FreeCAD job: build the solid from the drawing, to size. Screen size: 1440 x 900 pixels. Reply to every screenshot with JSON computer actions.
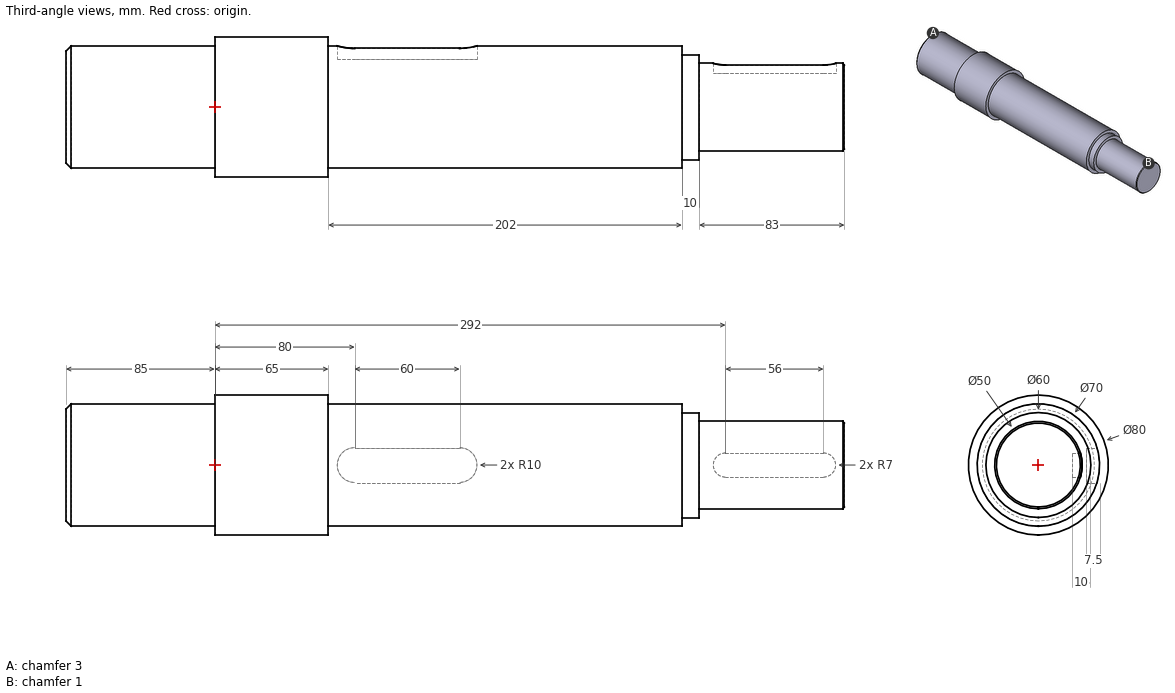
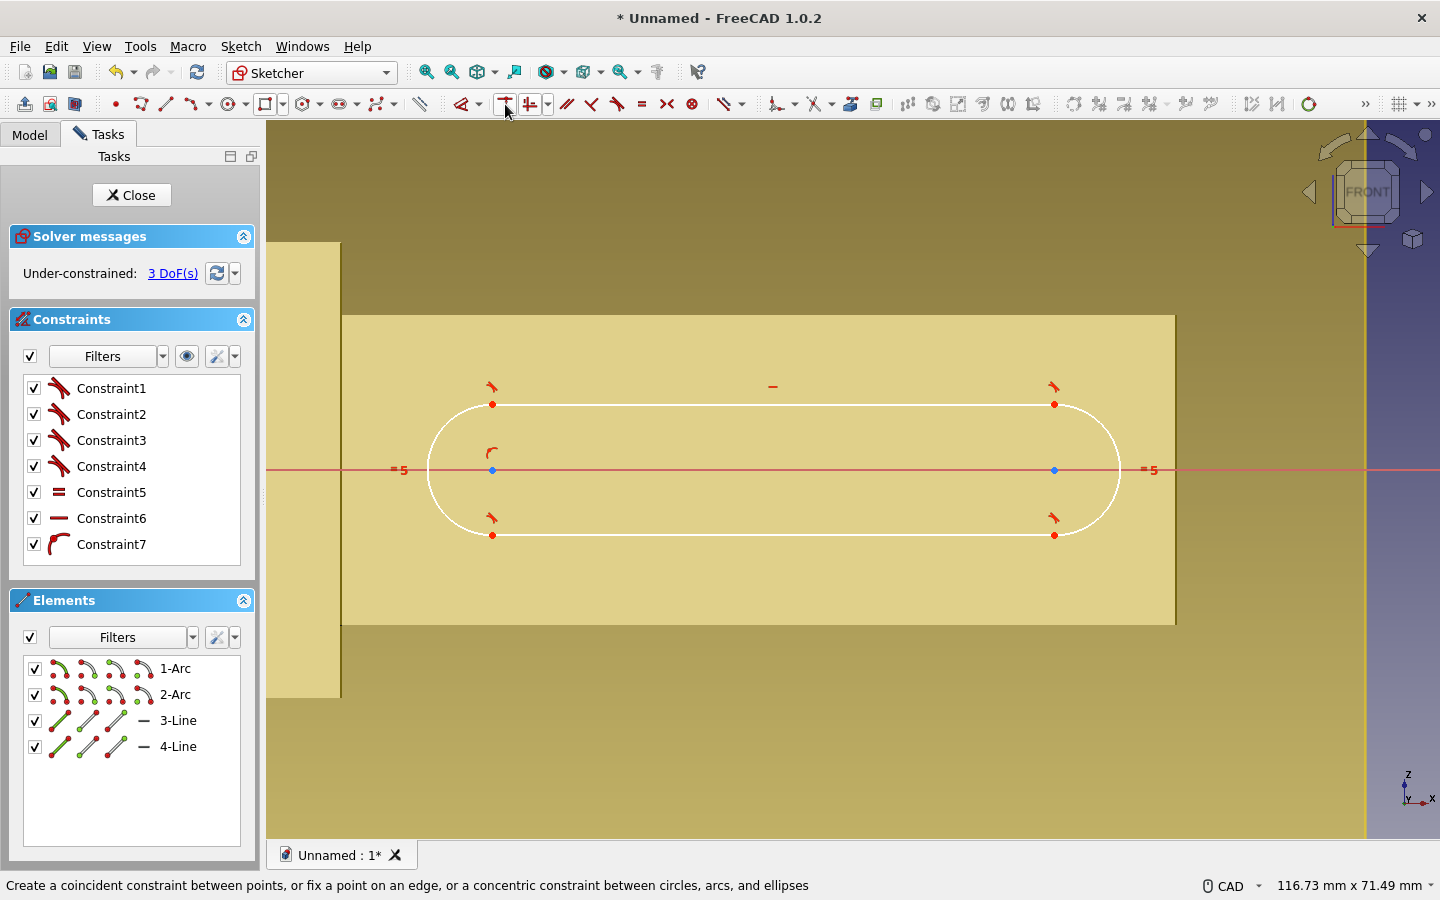
{"action": "left_click", "coordinate": [440, 432]}
{"action": "left_click", "coordinate": [414, 413]}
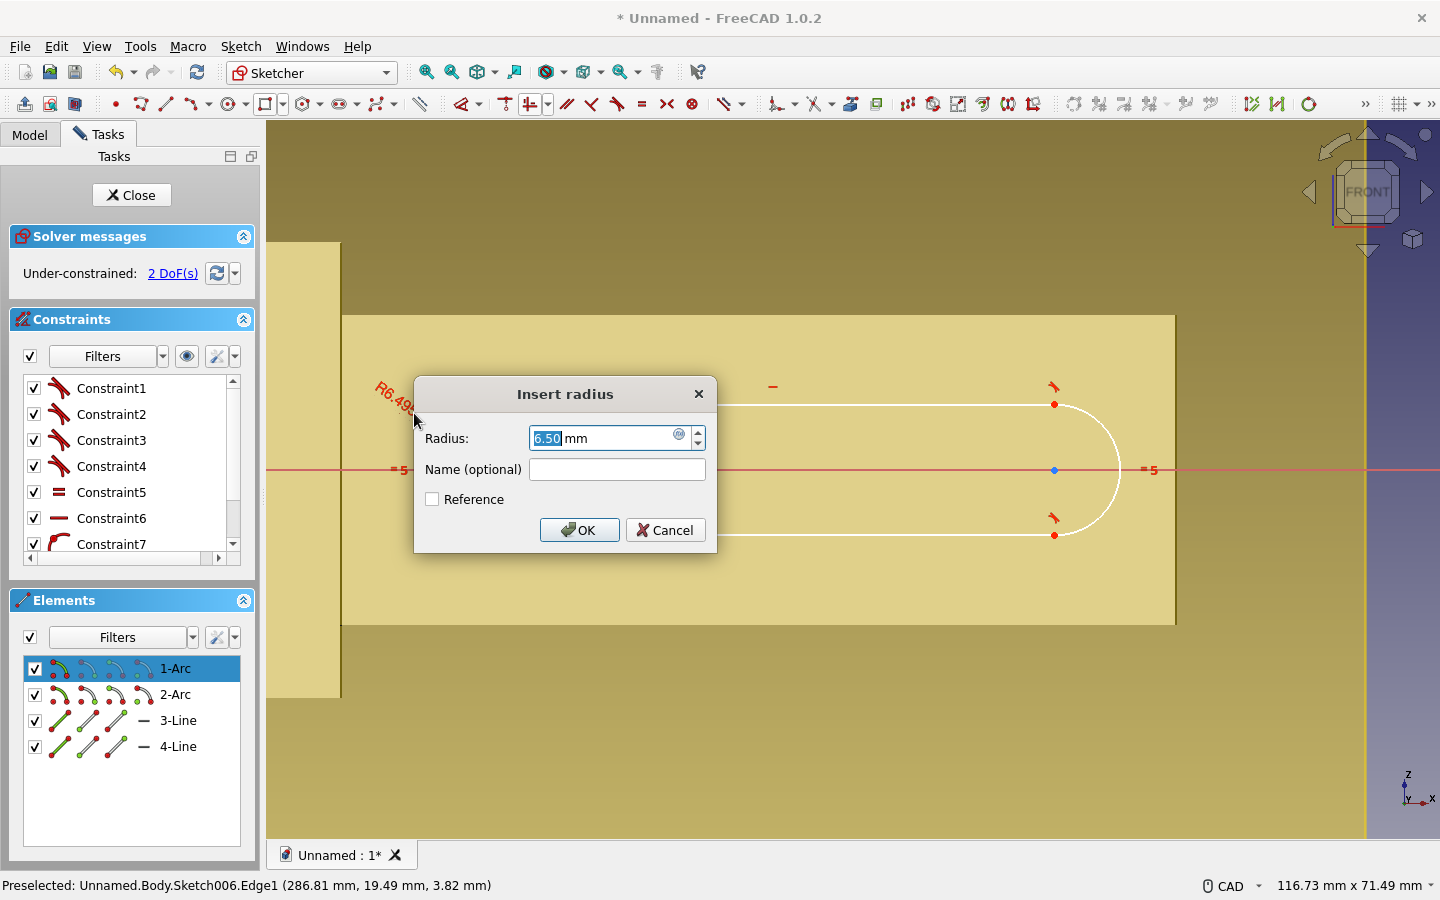
{"action": "type", "text": "7"}
{"action": "key", "text": "Return"}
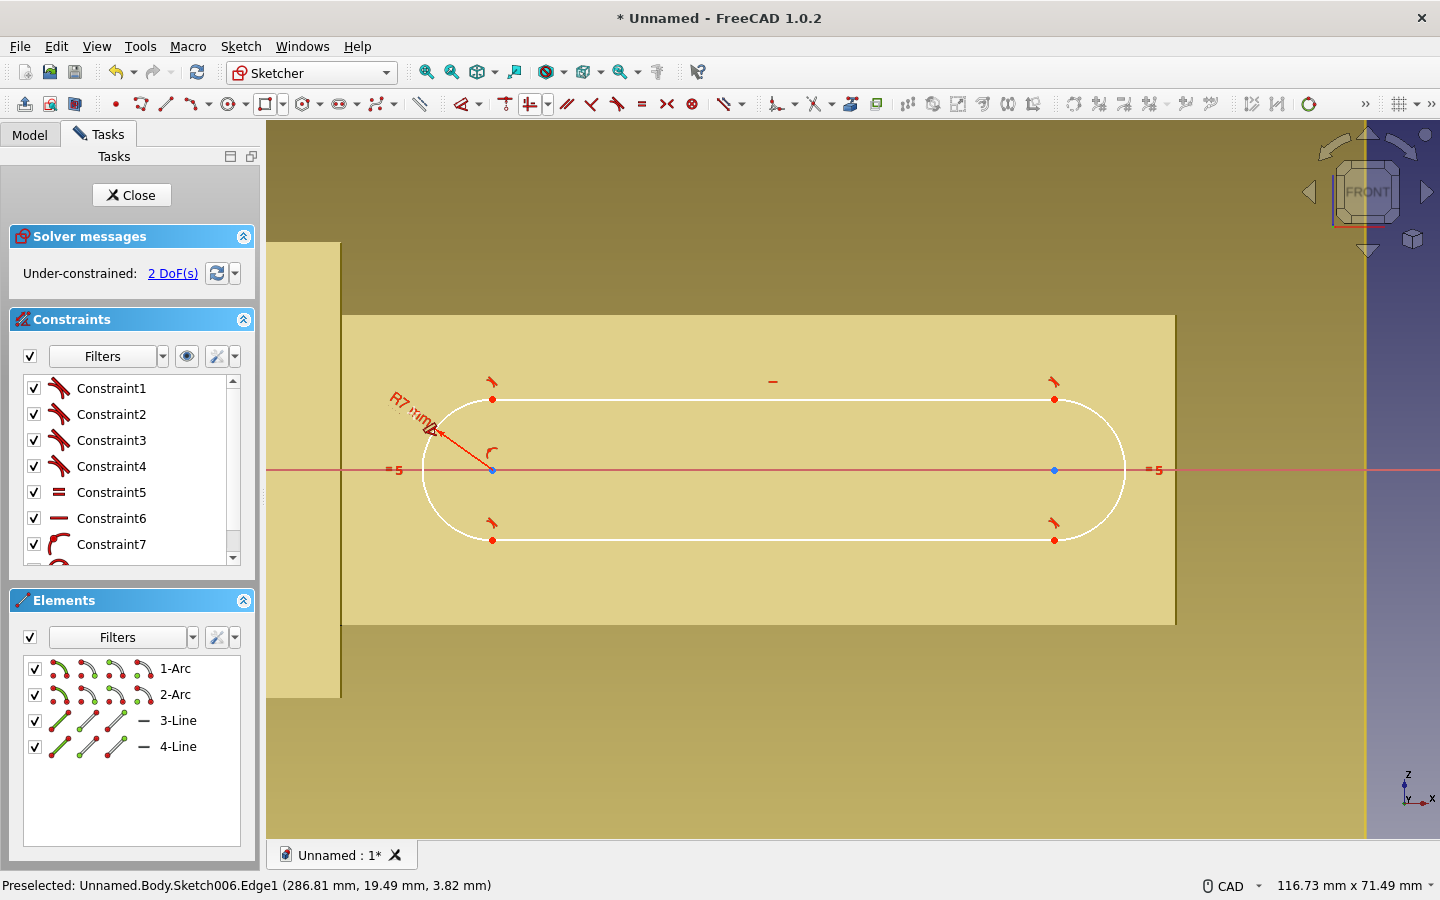
{"action": "left_click", "coordinate": [661, 400]}
{"action": "left_click", "coordinate": [774, 366]}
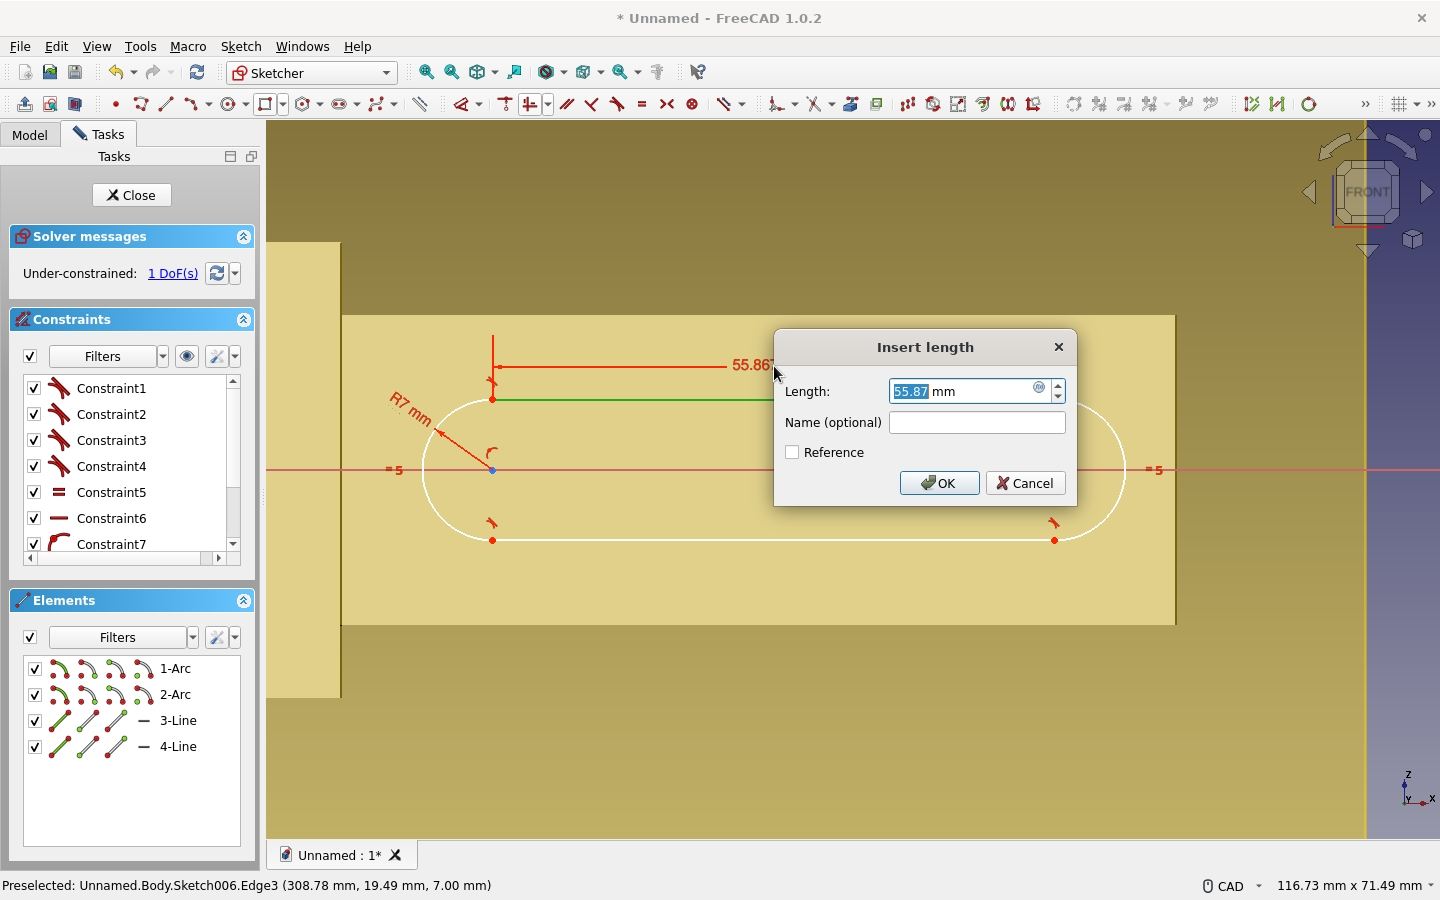
{"action": "type", "text": "56"}
{"action": "key", "text": "Return"}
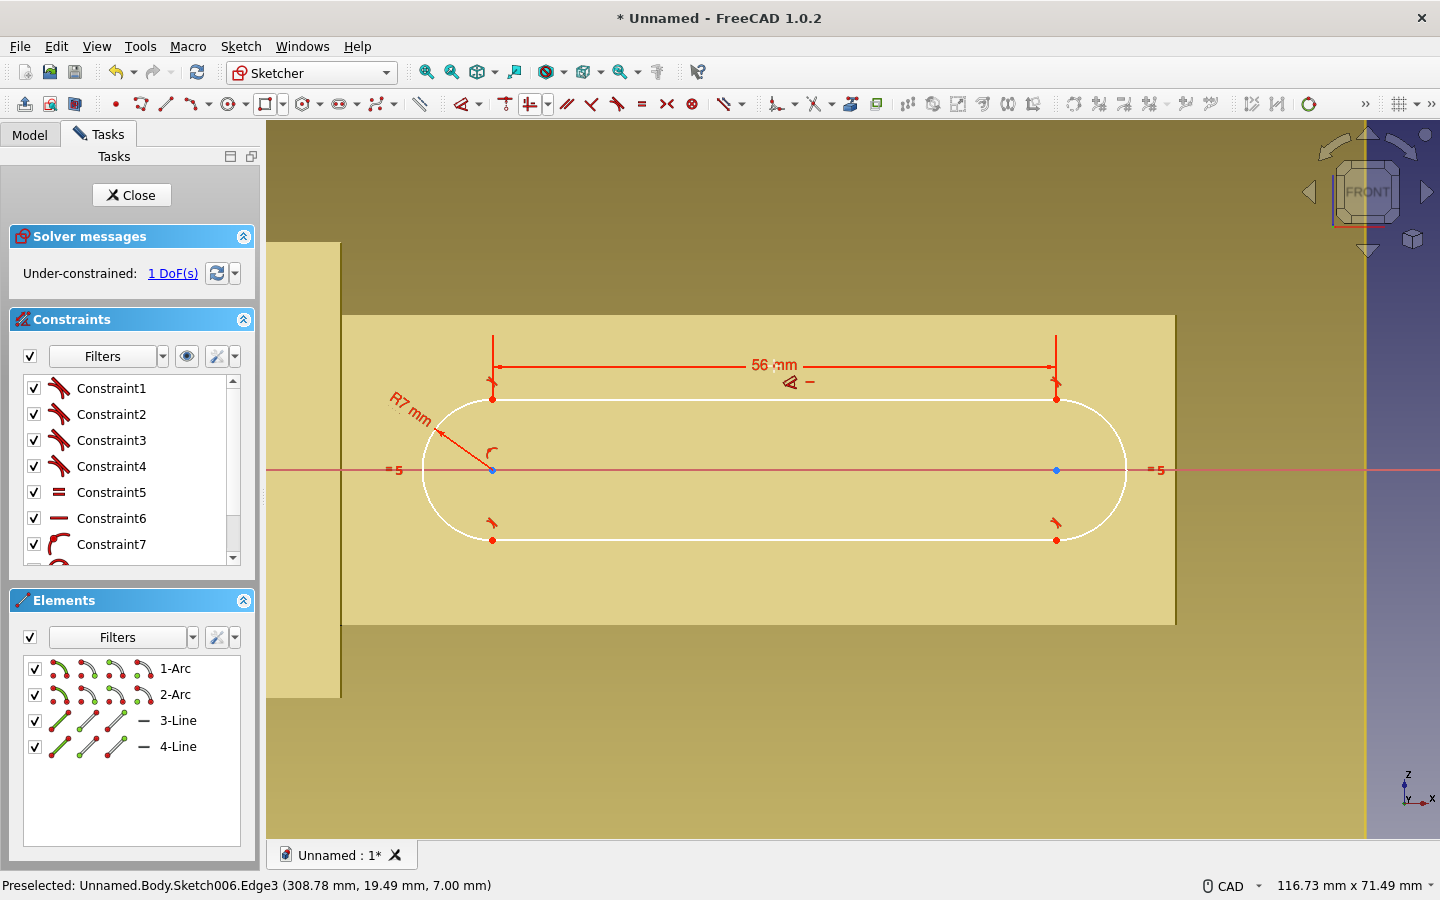
{"action": "left_click", "coordinate": [493, 400]}
{"action": "left_click", "coordinate": [393, 366]}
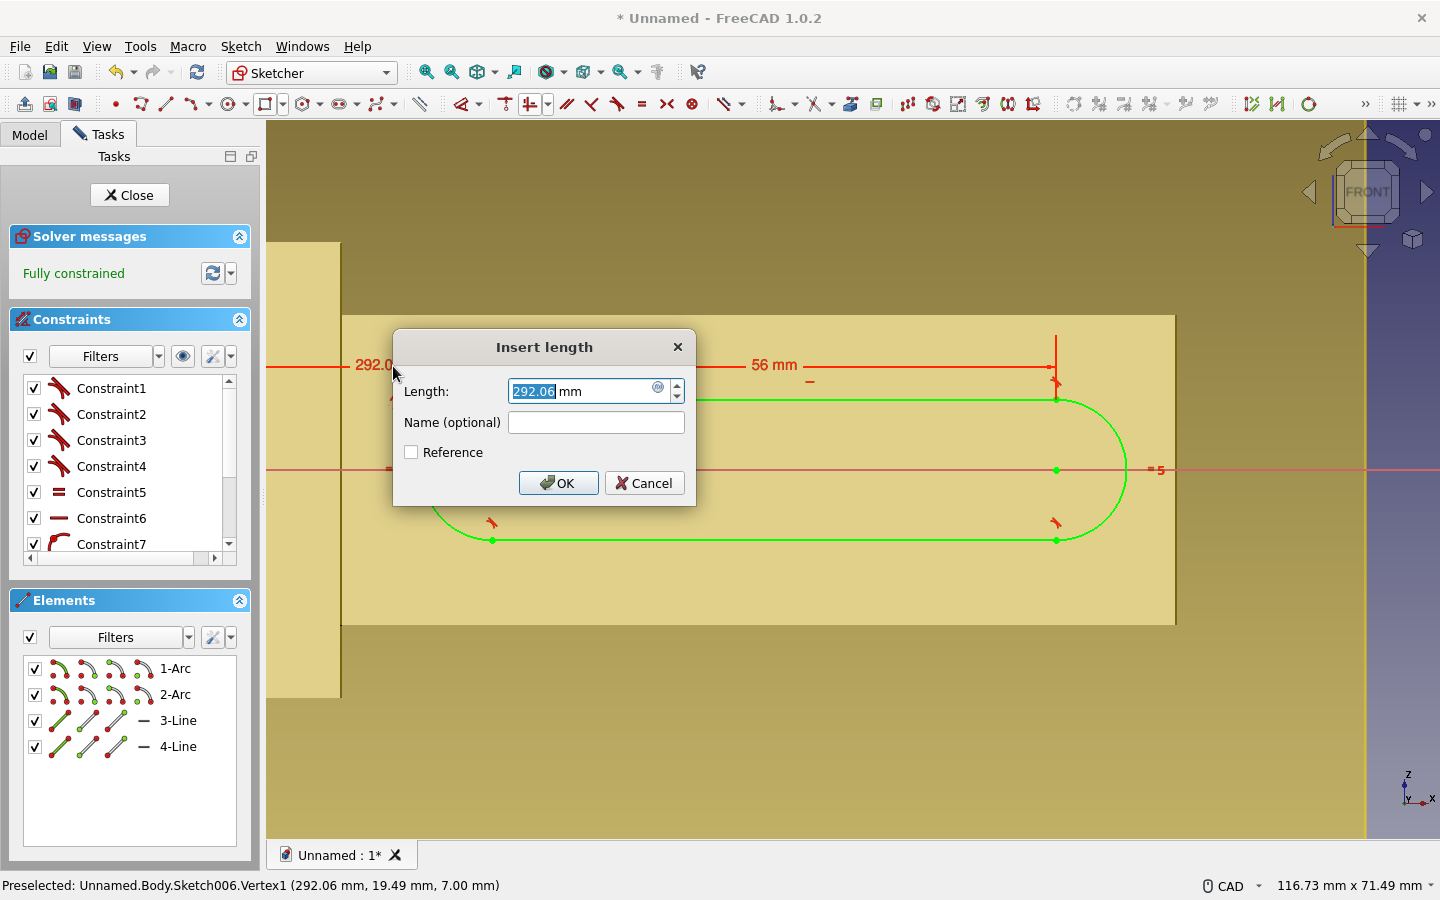
{"action": "type", "text": "292"}
{"action": "key", "text": "Return"}
{"action": "key", "text": "Escape"}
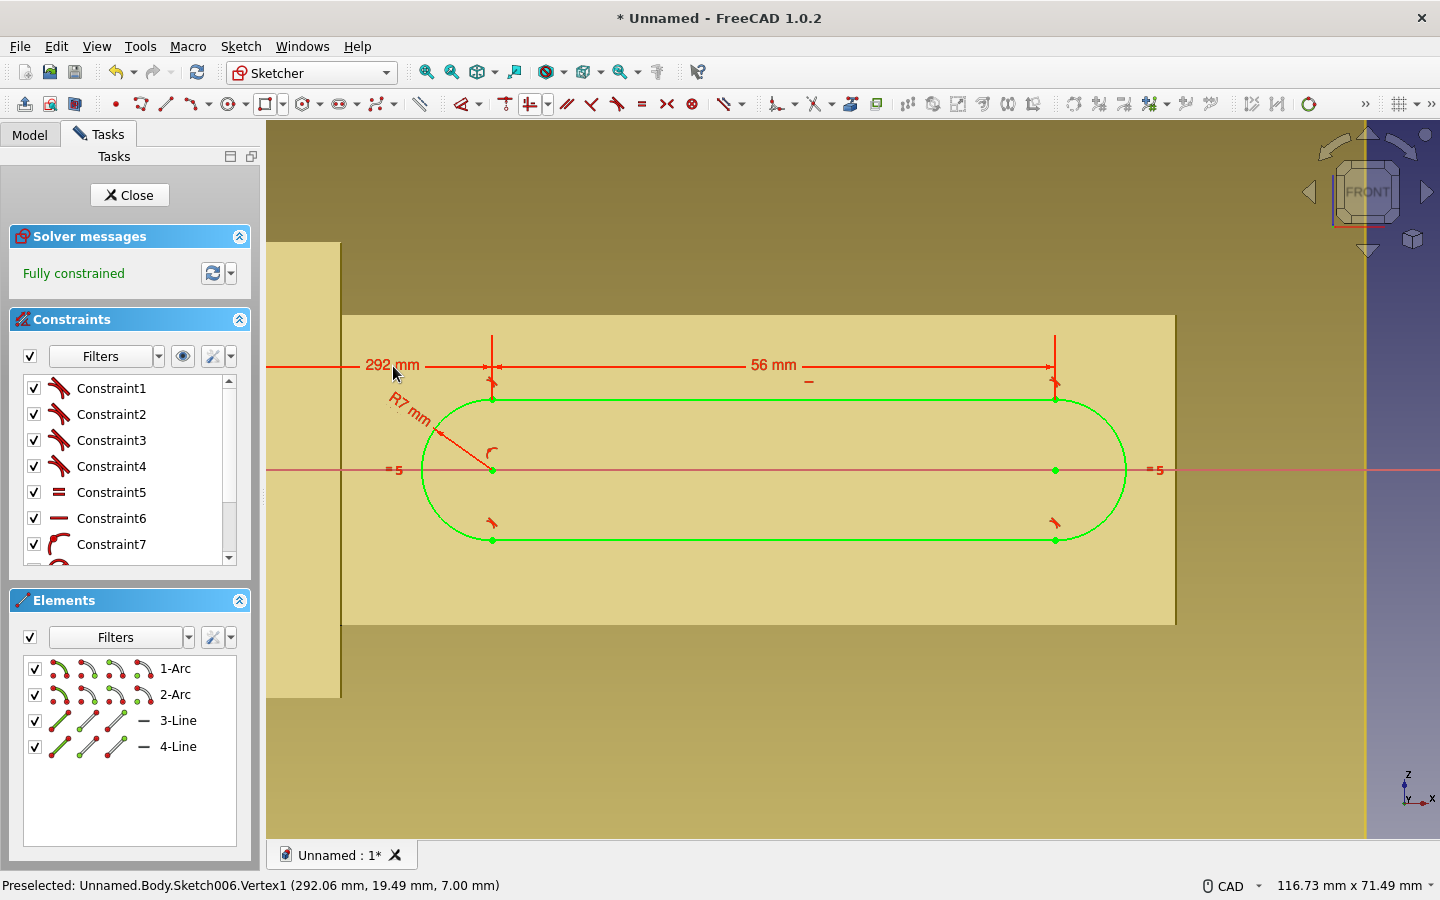
{"action": "left_click", "coordinate": [130, 195]}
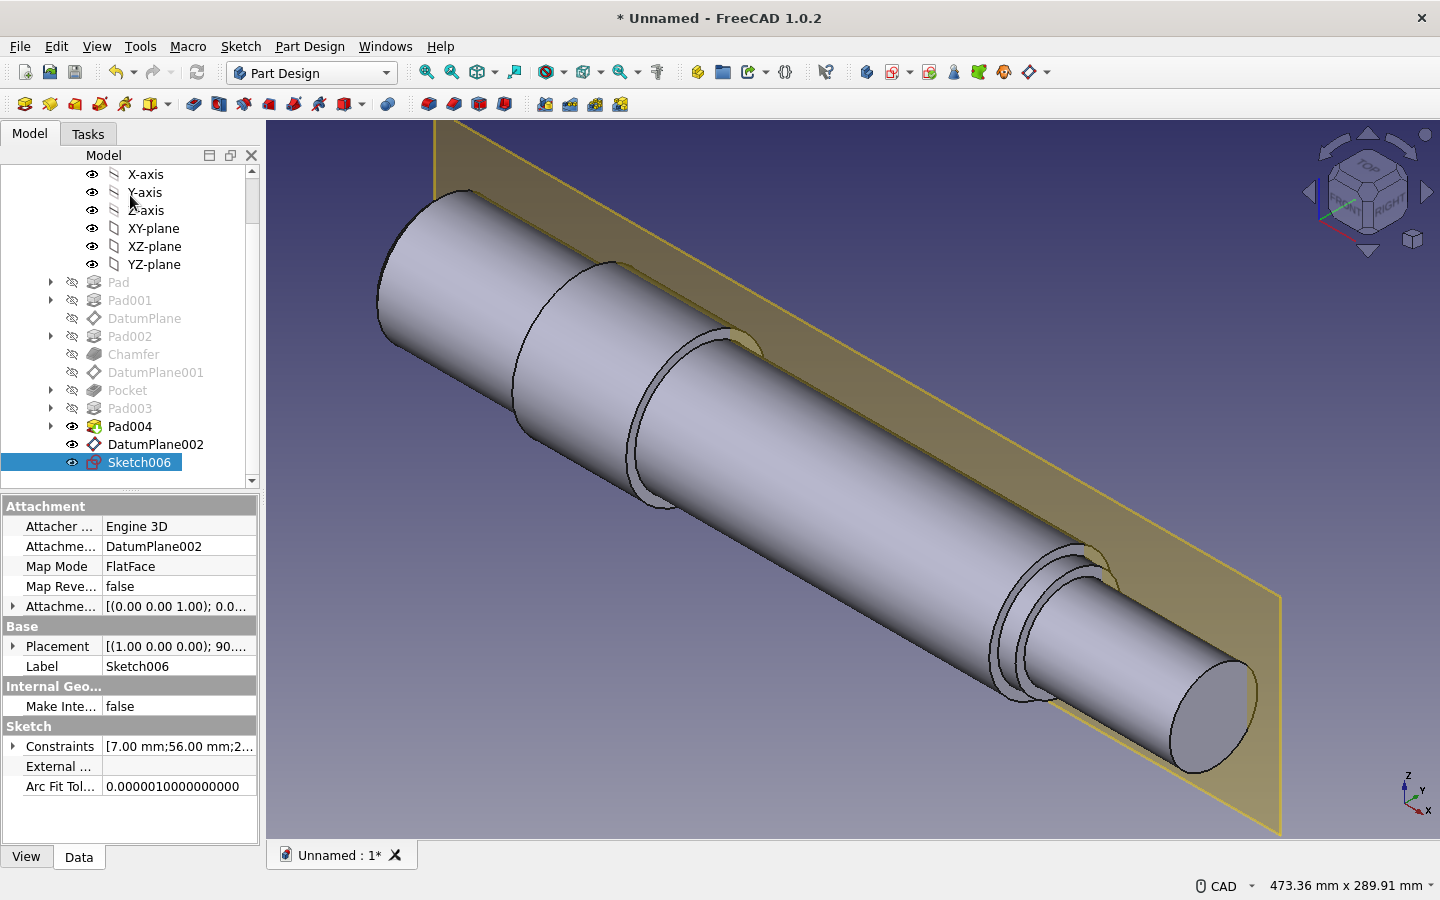
{"action": "left_click", "coordinate": [194, 104]}